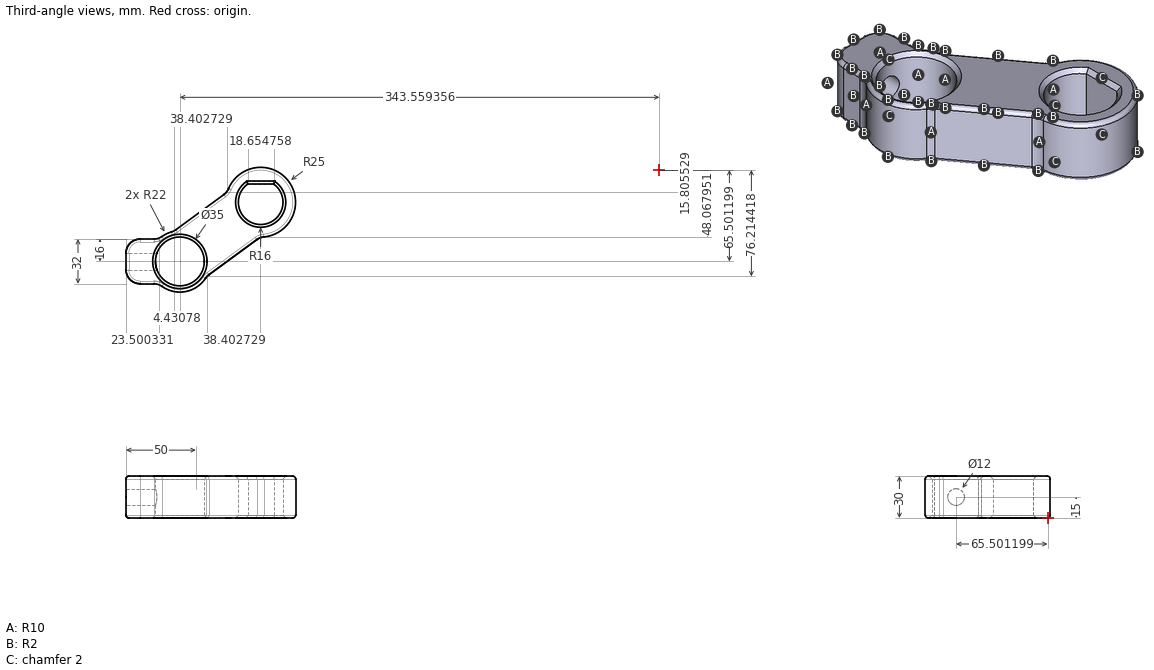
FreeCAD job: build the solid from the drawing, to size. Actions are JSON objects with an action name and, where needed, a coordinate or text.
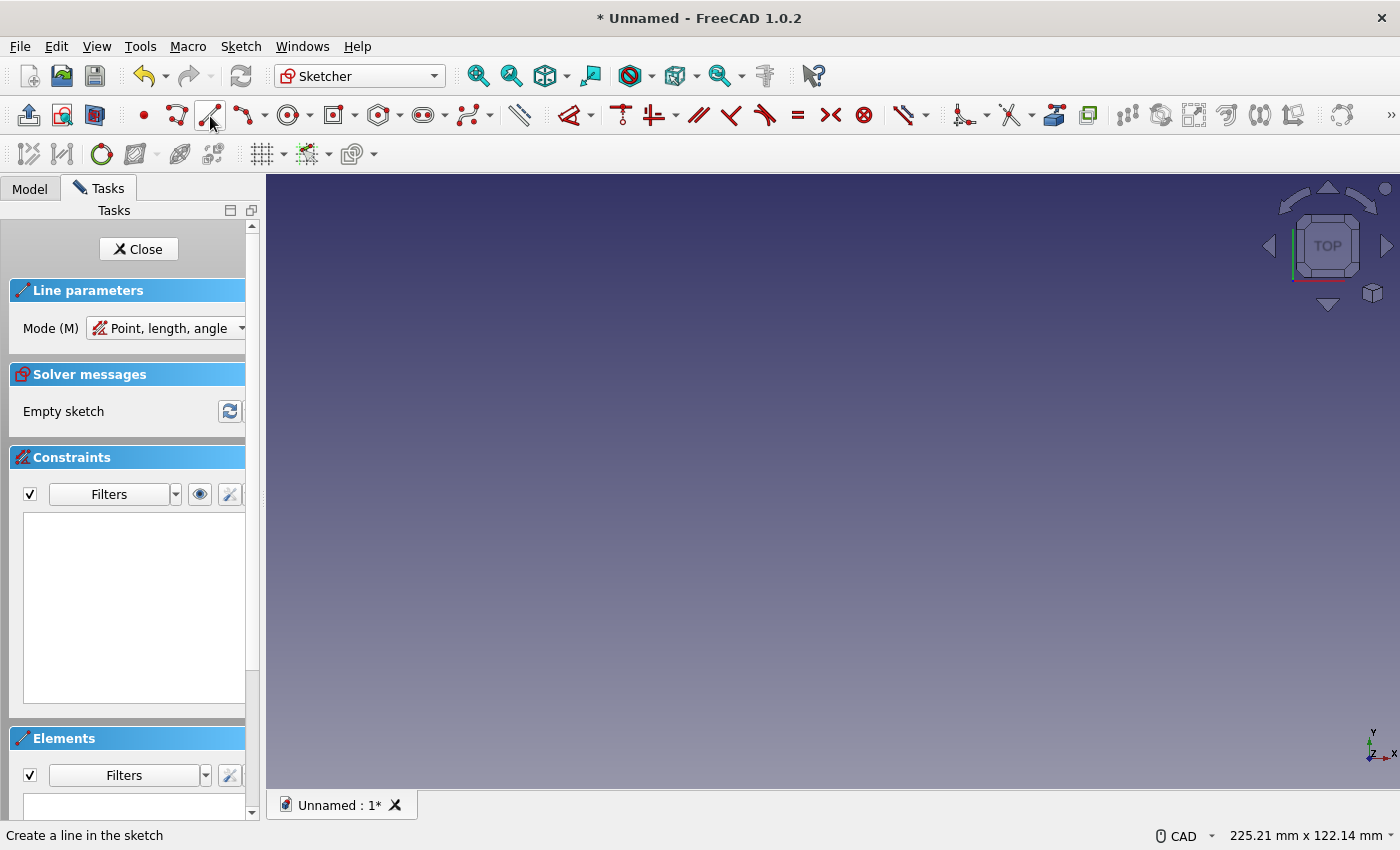
{"action": "left_click", "coordinate": [834, 318]}
{"action": "left_click", "coordinate": [640, 460]}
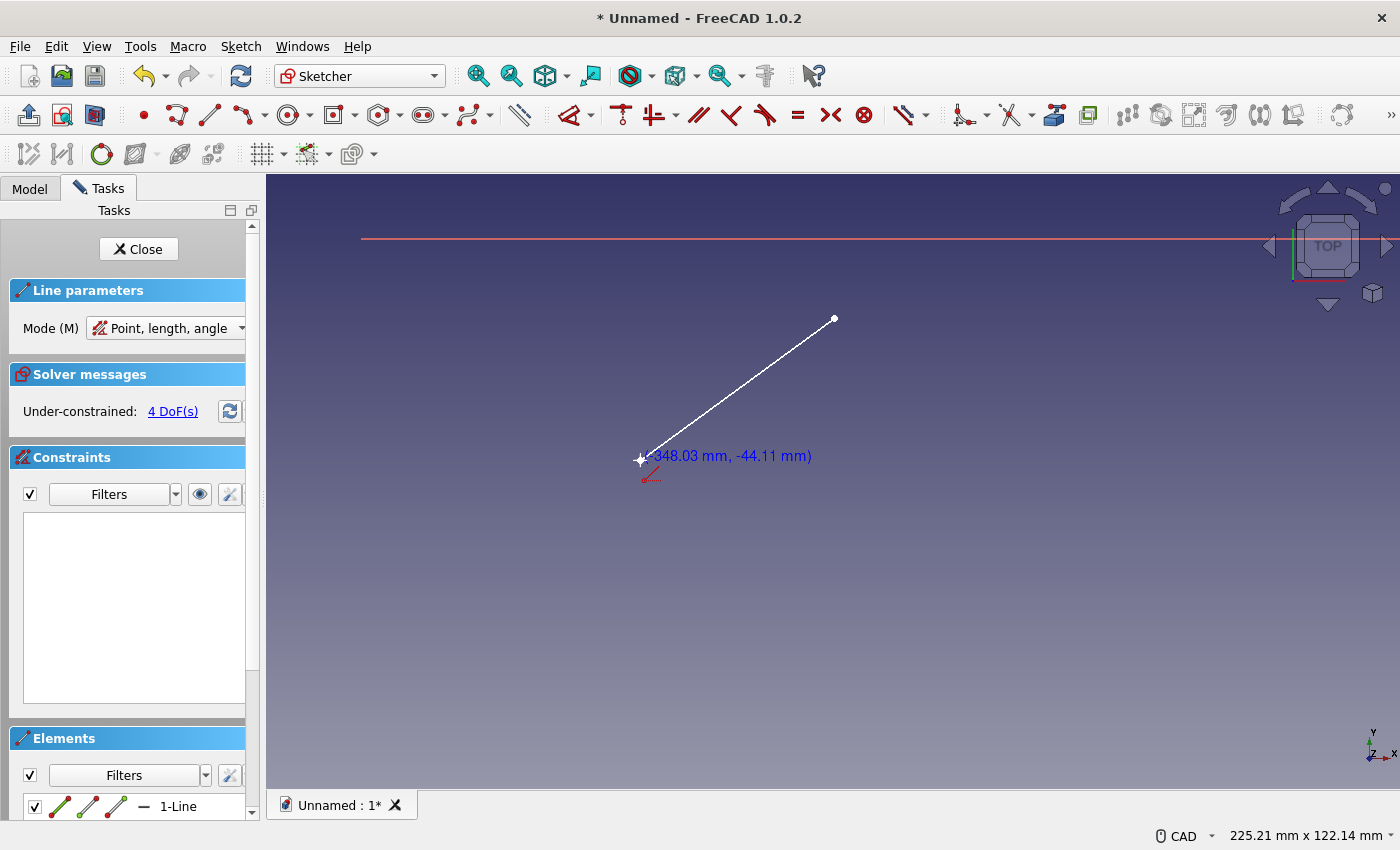
{"action": "left_click", "coordinate": [177, 116]}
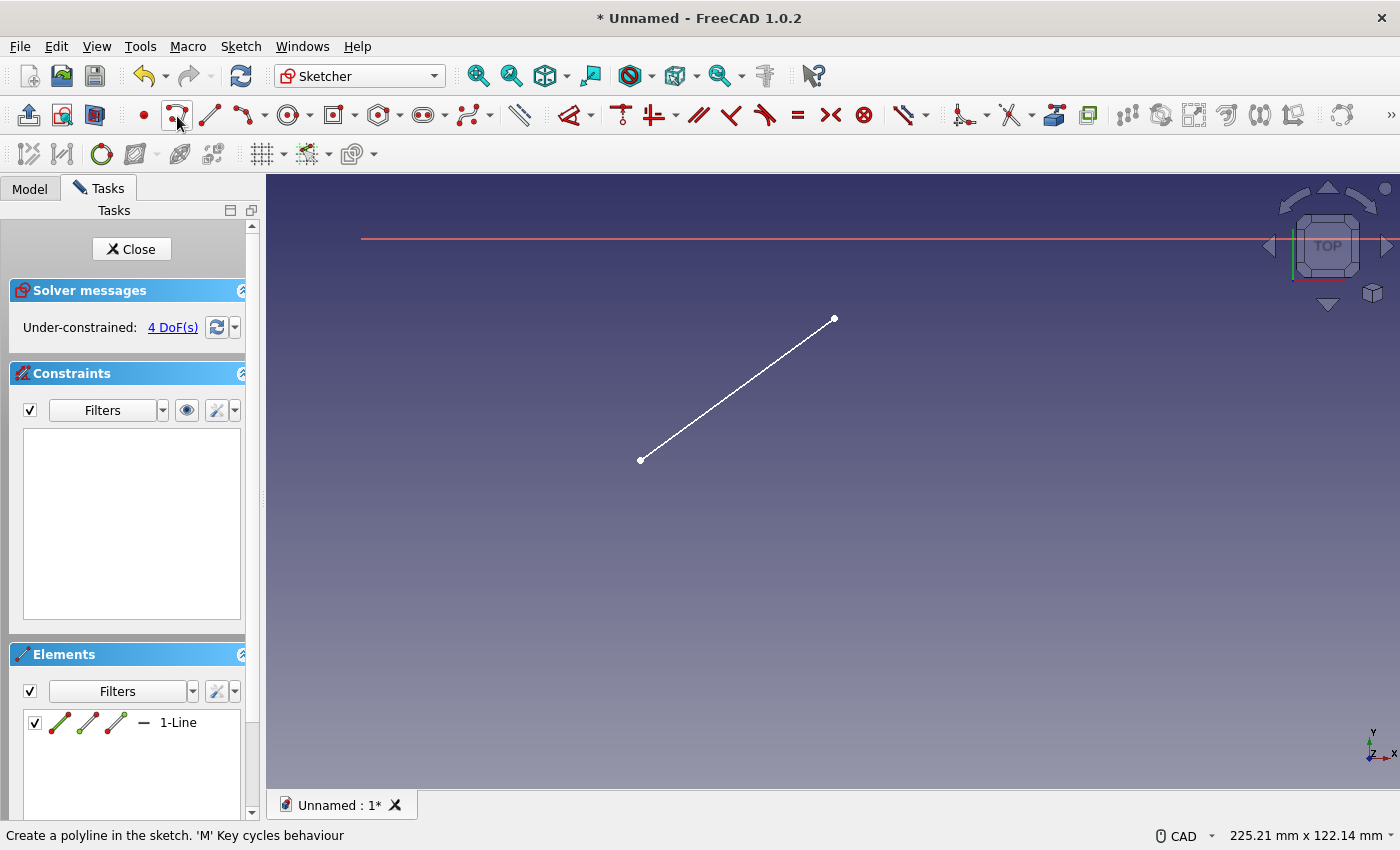
{"action": "left_click", "coordinate": [586, 488]}
{"action": "left_click", "coordinate": [468, 488]}
{"action": "left_click", "coordinate": [468, 649]}
{"action": "left_click", "coordinate": [586, 649]}
{"action": "right_click", "coordinate": [586, 649]}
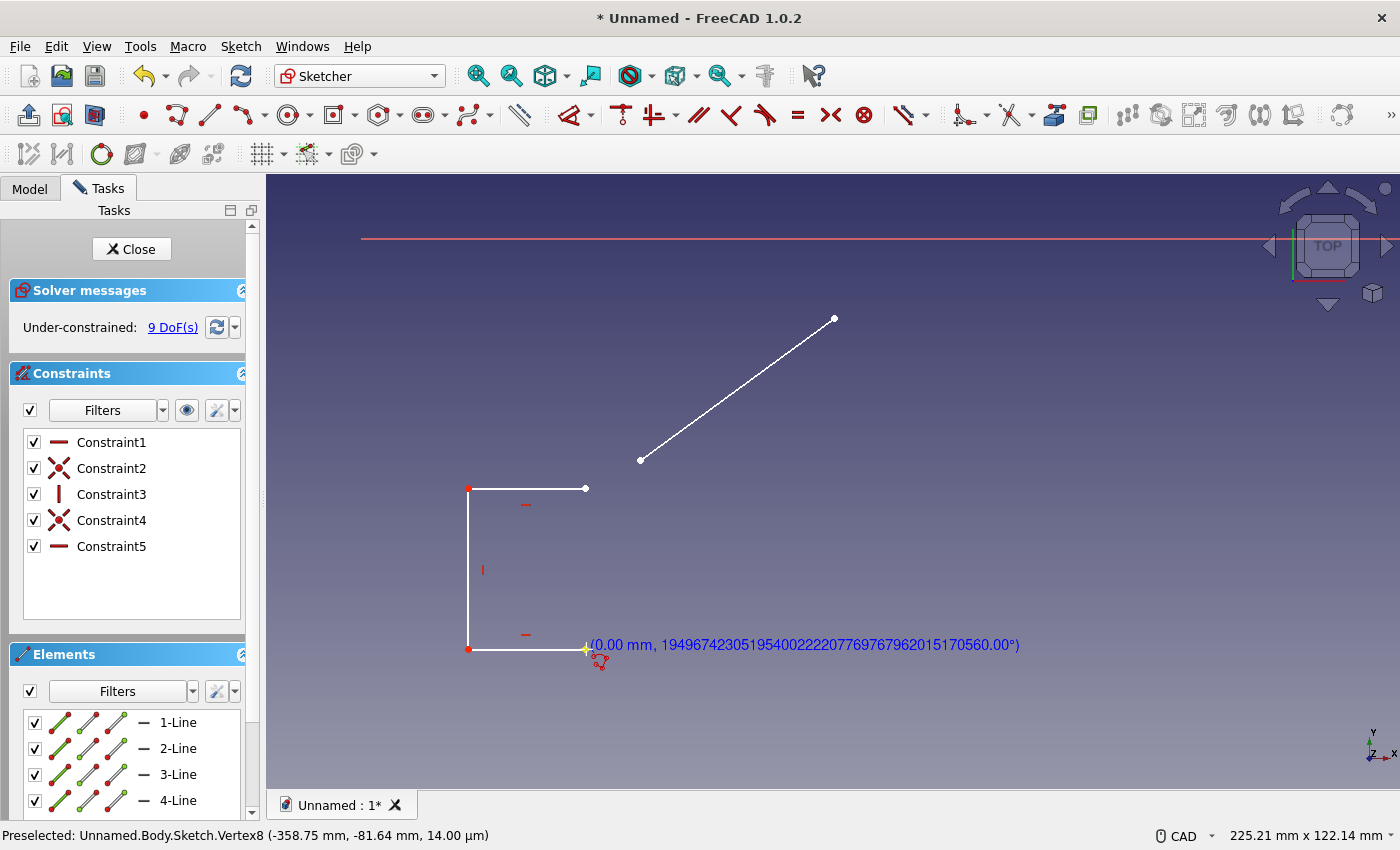
{"action": "key", "text": "g l"}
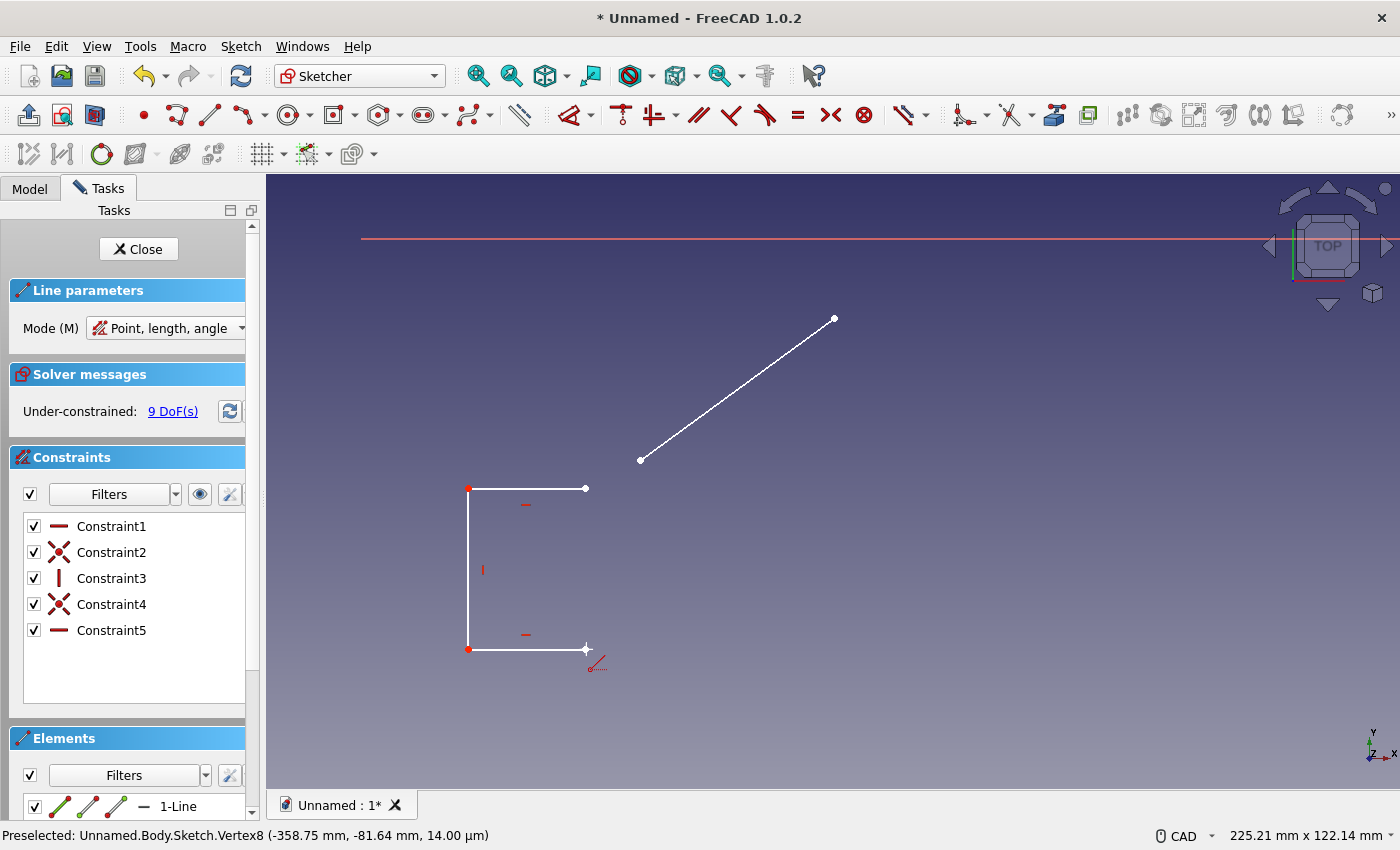
{"action": "left_click", "coordinate": [759, 623]}
{"action": "left_click", "coordinate": [953, 481]}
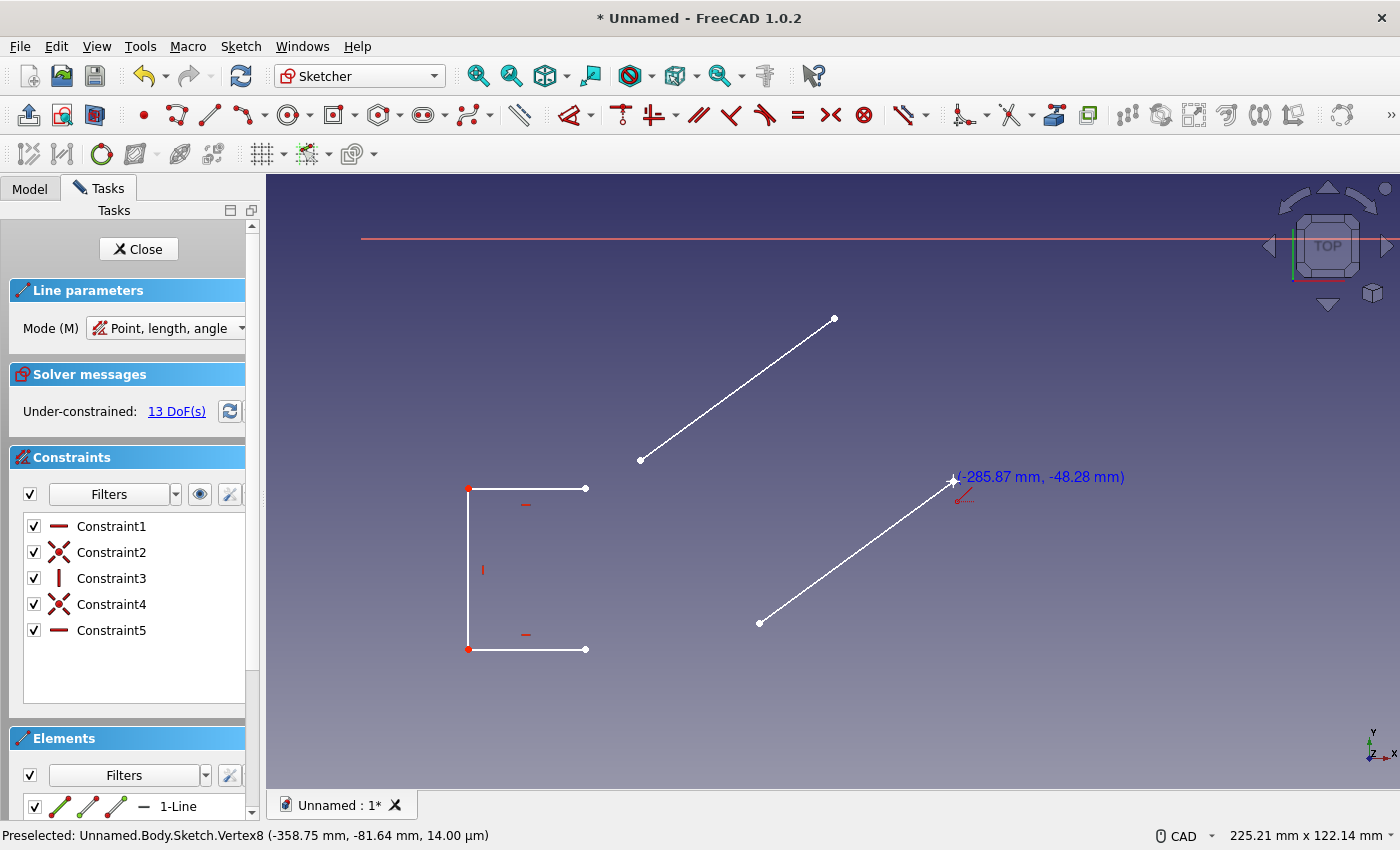
{"action": "left_click", "coordinate": [242, 116]}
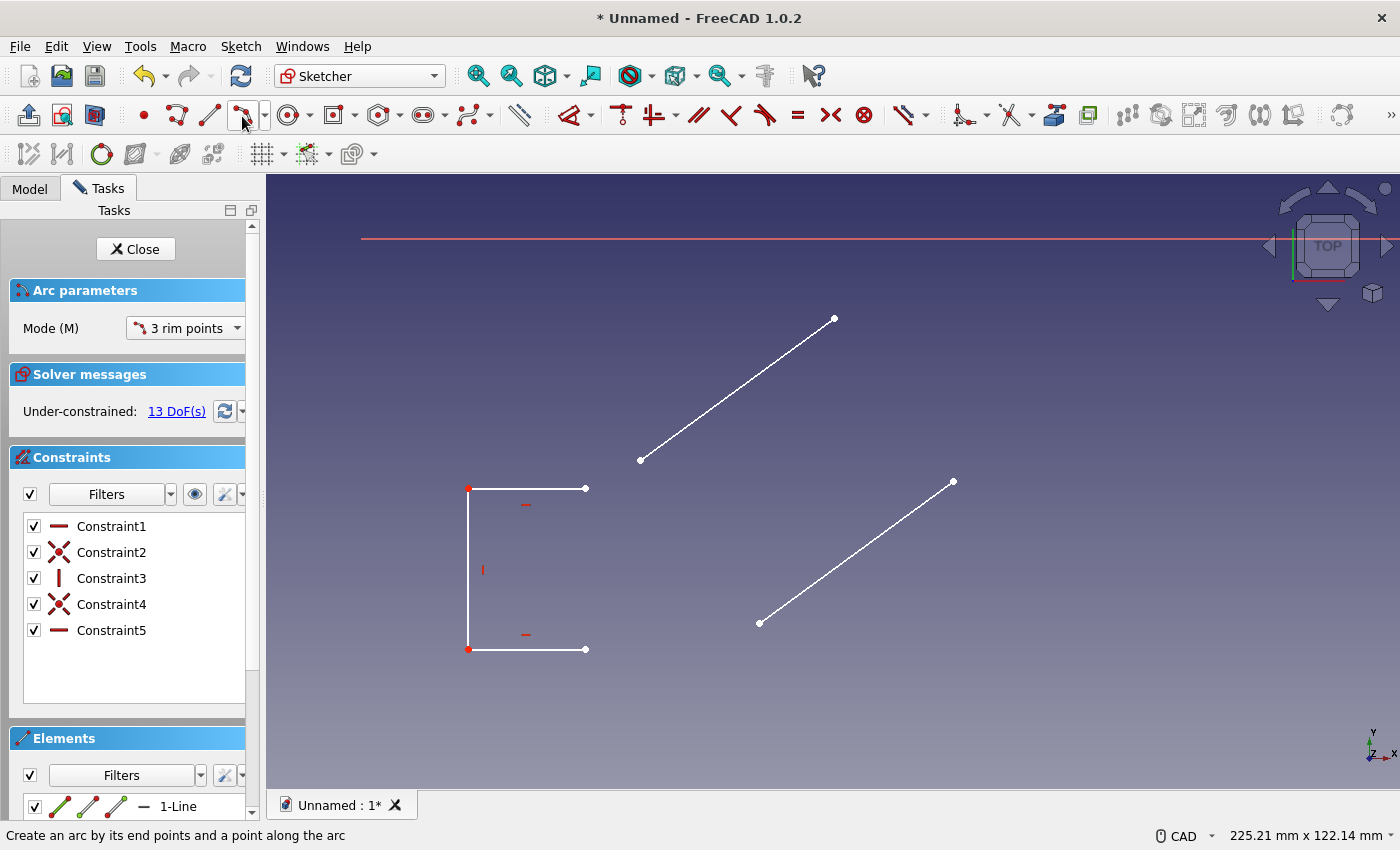
{"action": "left_click", "coordinate": [640, 461]}
{"action": "left_click", "coordinate": [586, 489]}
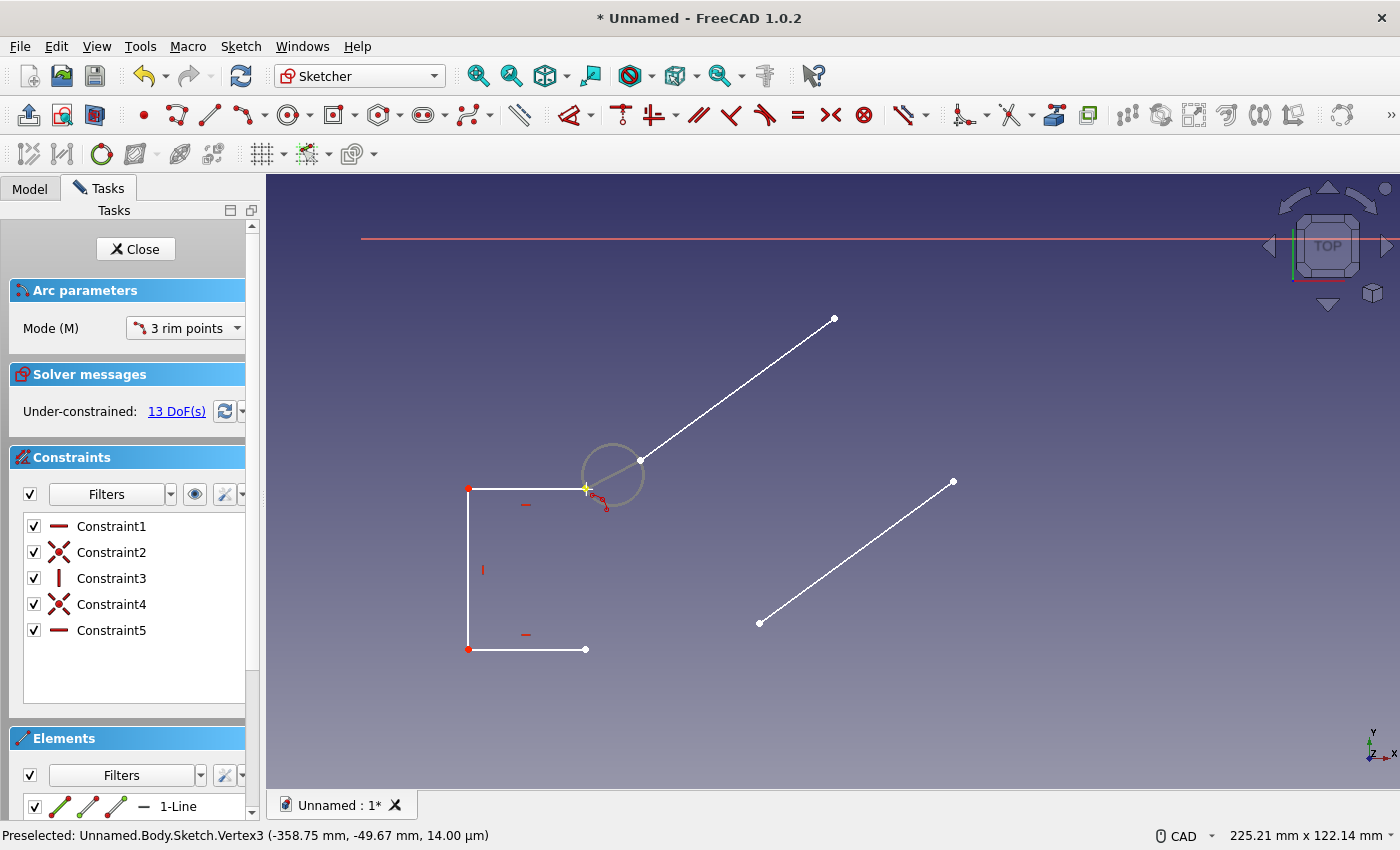
{"action": "scroll", "coordinate": [611, 470], "scroll_direction": "up", "scroll_amount": 7}